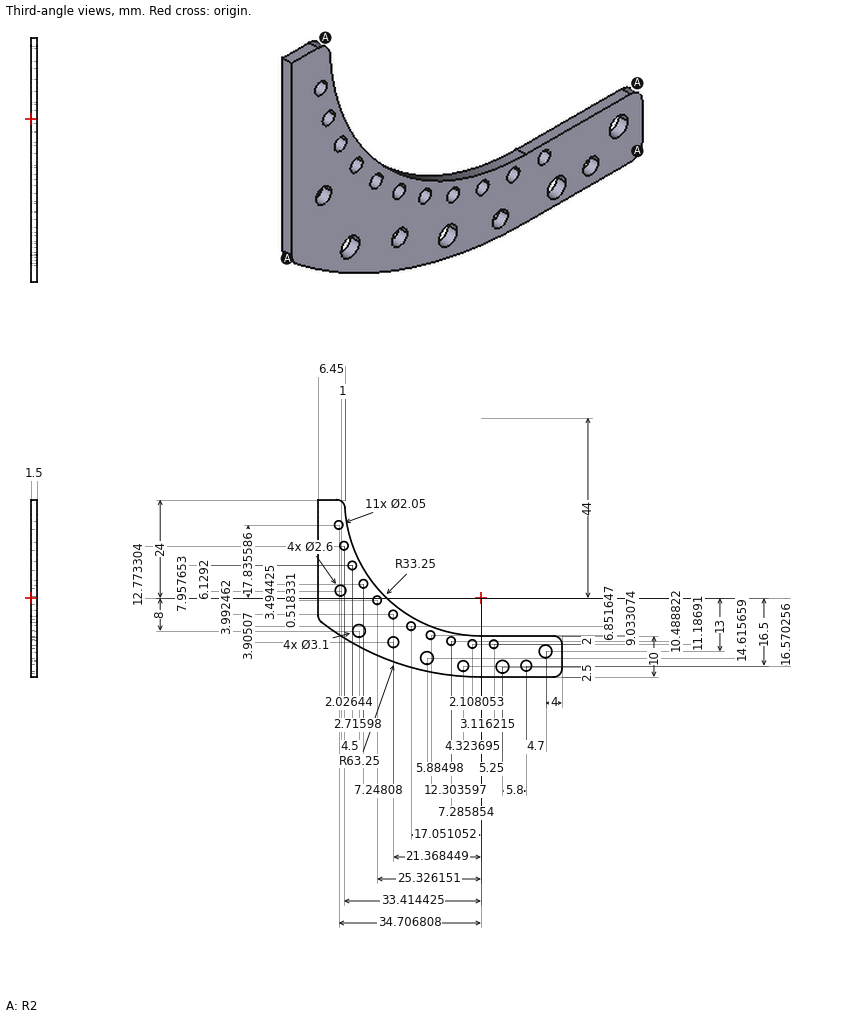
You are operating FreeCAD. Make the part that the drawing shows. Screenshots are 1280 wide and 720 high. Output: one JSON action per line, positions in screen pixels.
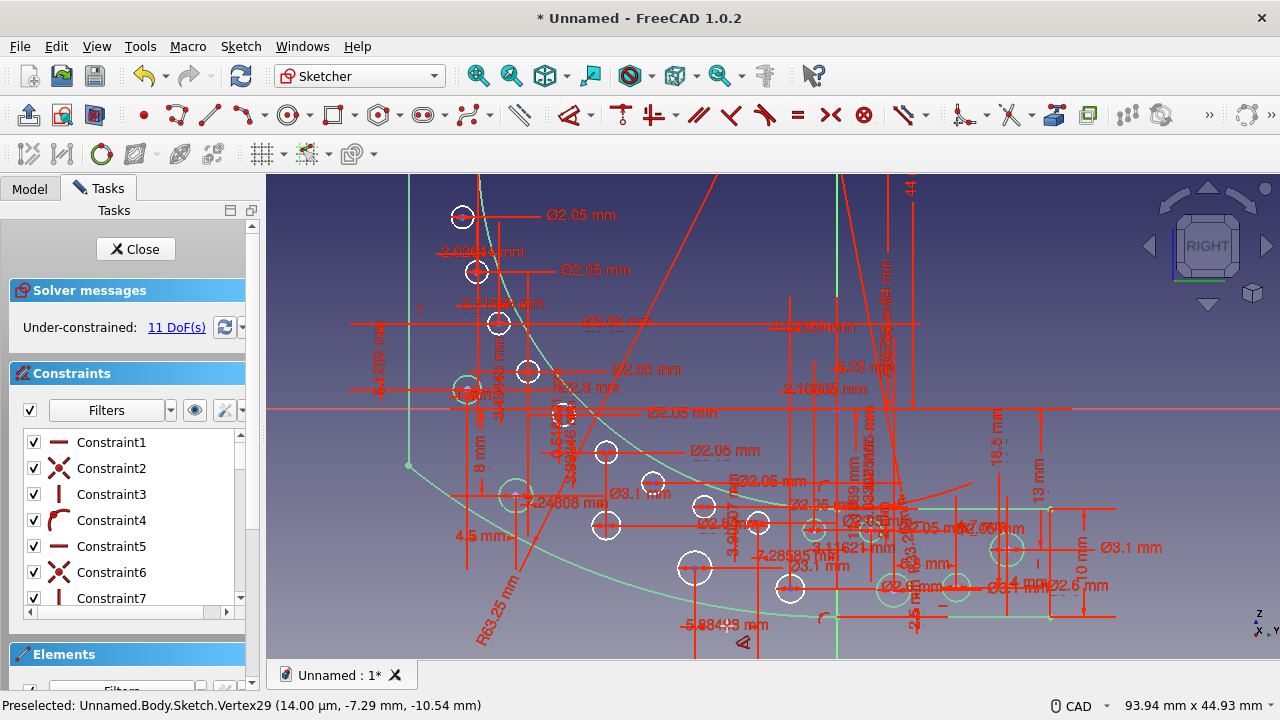
{"action": "left_click", "coordinate": [463, 217]}
{"action": "left_click", "coordinate": [736, 443]}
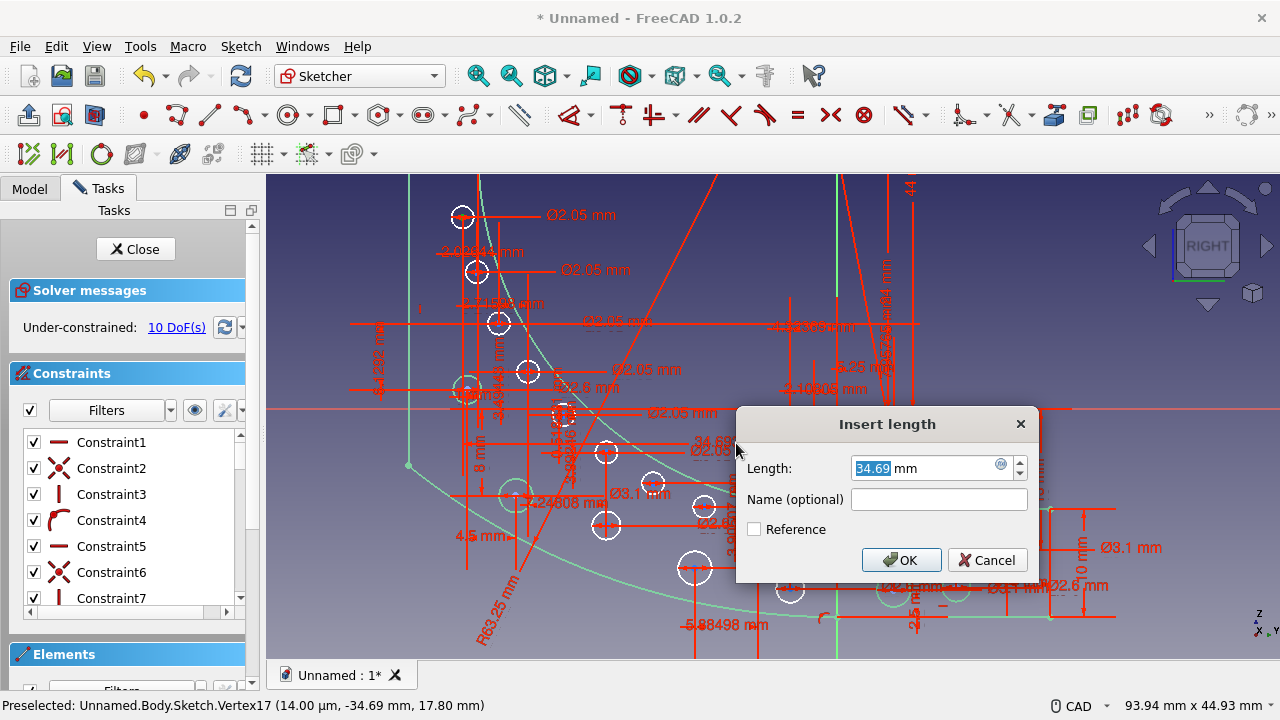
{"action": "type", "text": "34.706808"}
{"action": "key", "text": "Return"}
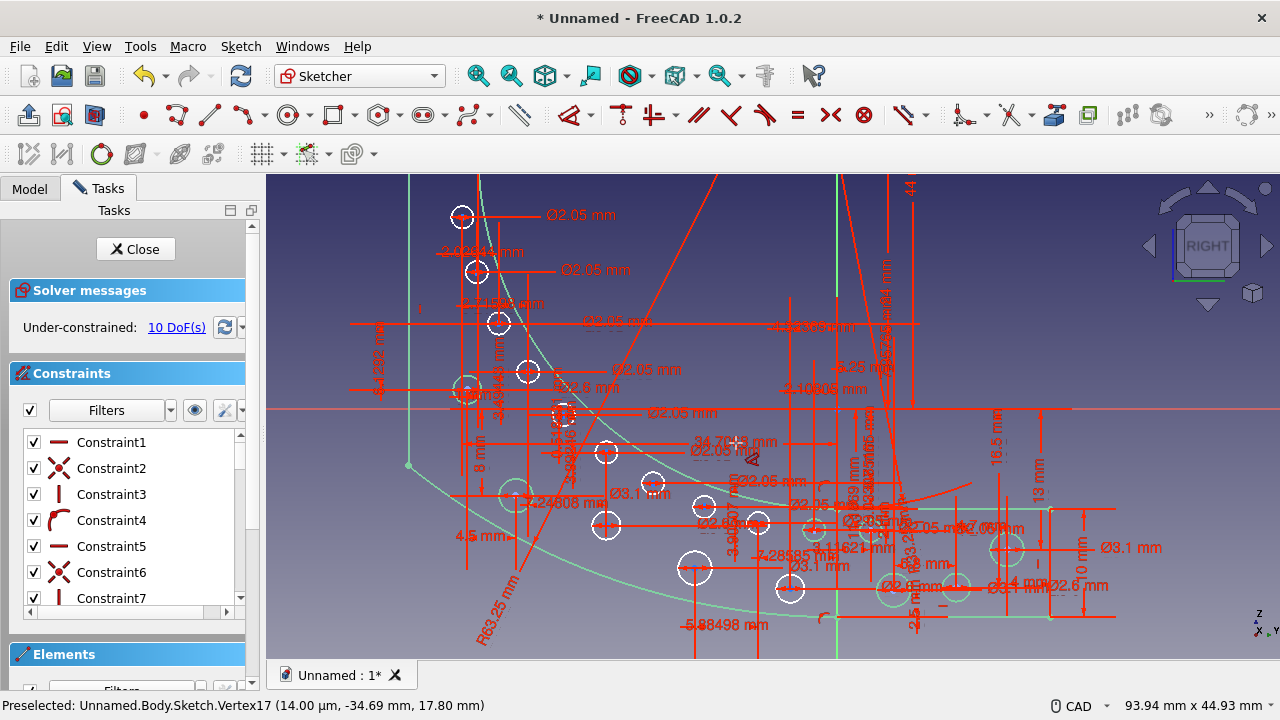
{"action": "left_click", "coordinate": [462, 217]}
{"action": "left_click", "coordinate": [428, 313]}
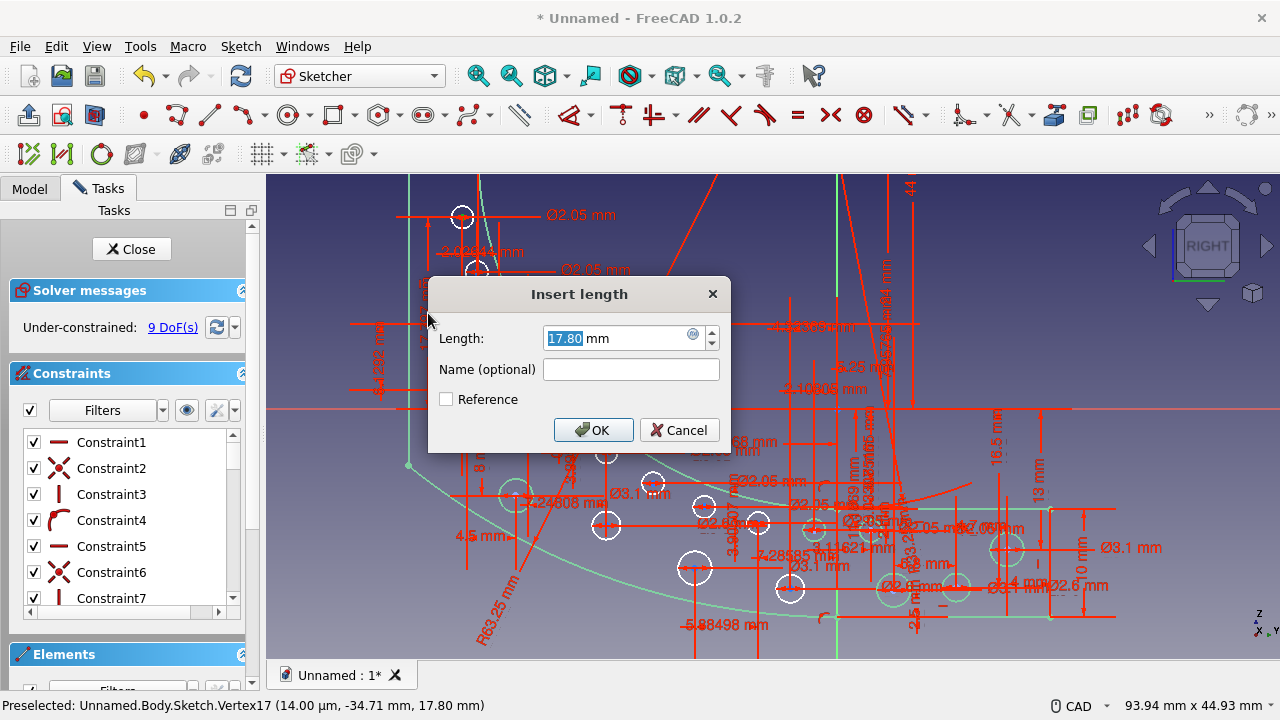
{"action": "type", "text": "17.835586"}
{"action": "key", "text": "Return"}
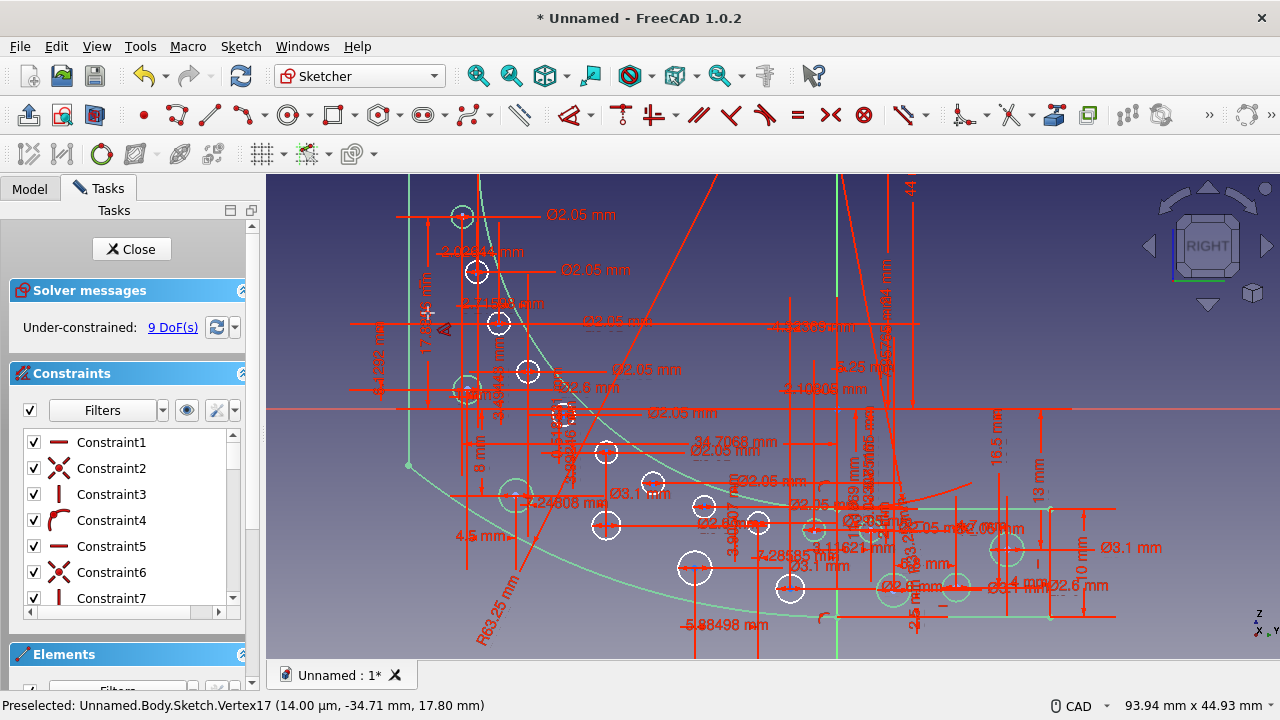
{"action": "left_click", "coordinate": [477, 272]}
{"action": "left_click", "coordinate": [657, 238]}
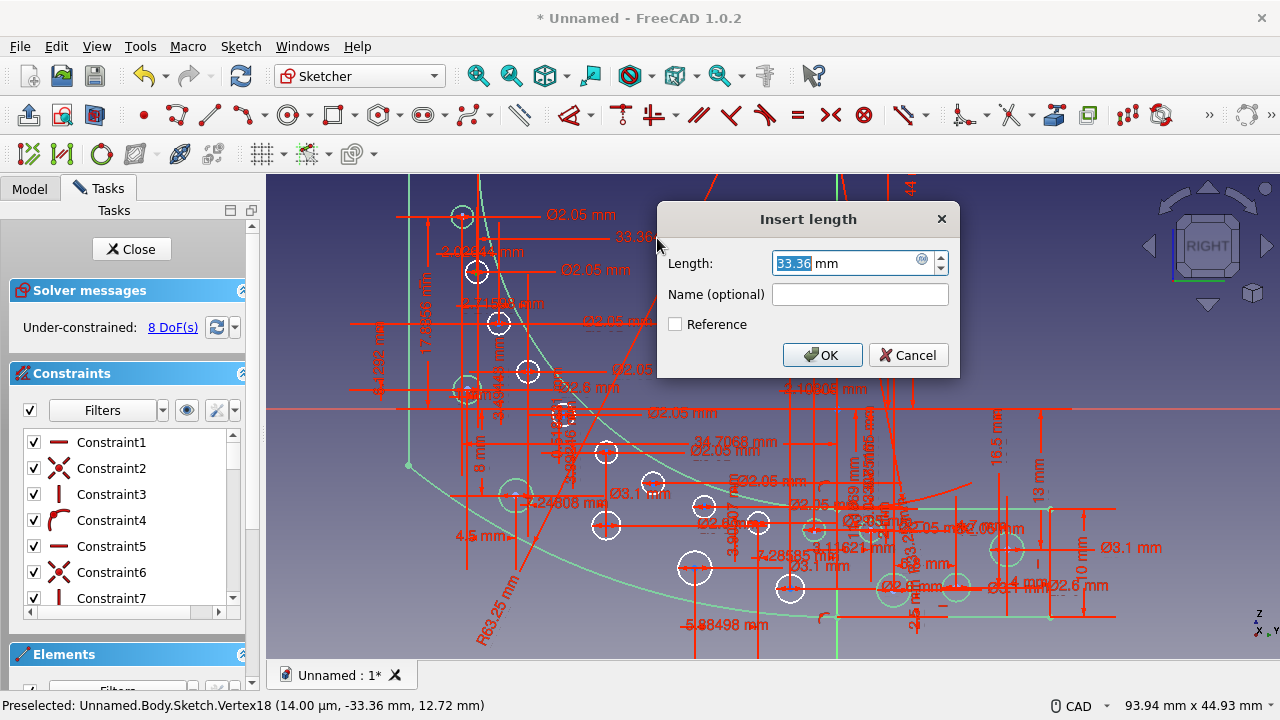
{"action": "type", "text": "33.414425"}
{"action": "key", "text": "Return"}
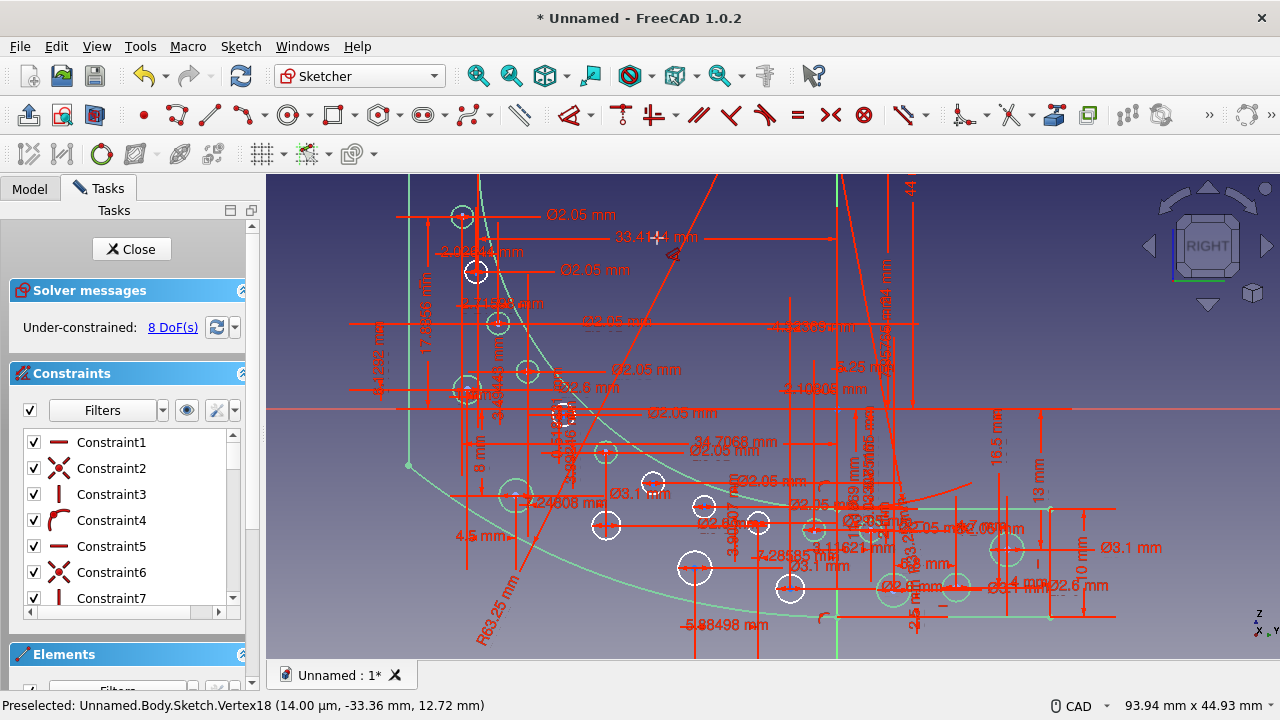
{"action": "left_click", "coordinate": [476, 272]}
{"action": "left_click", "coordinate": [895, 309]}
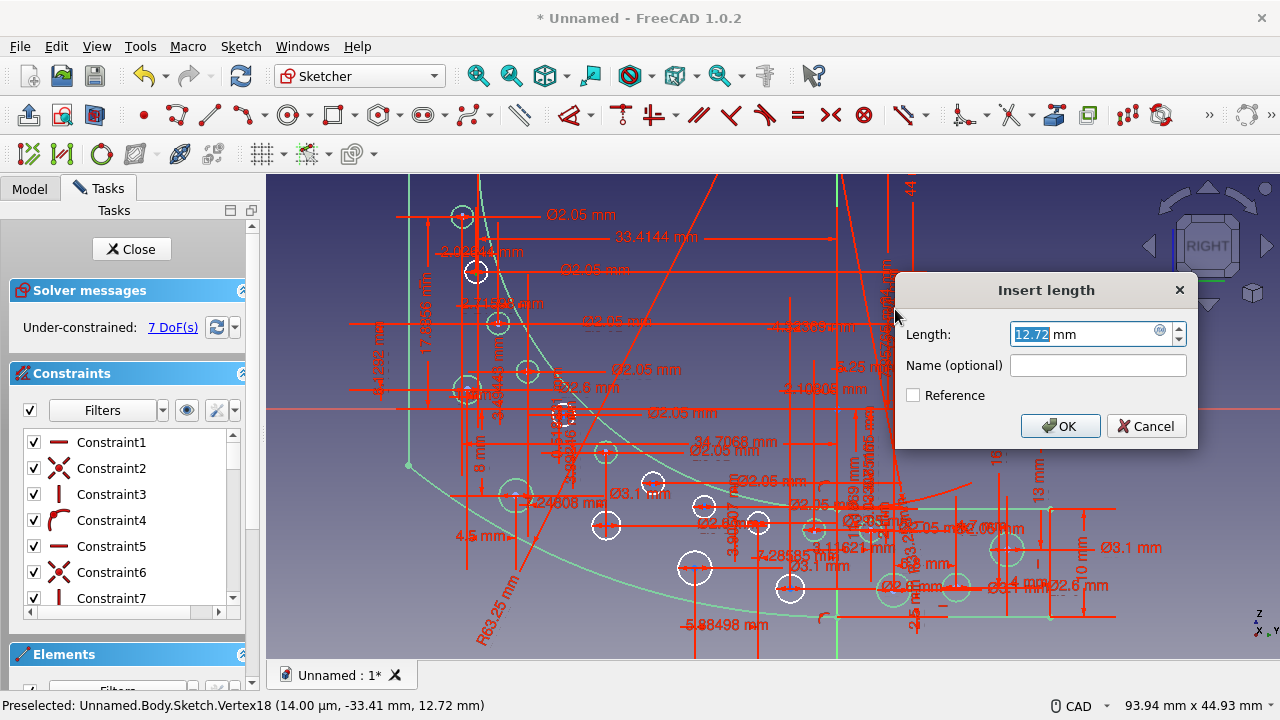
{"action": "type", "text": "12.773304"}
{"action": "key", "text": "Return"}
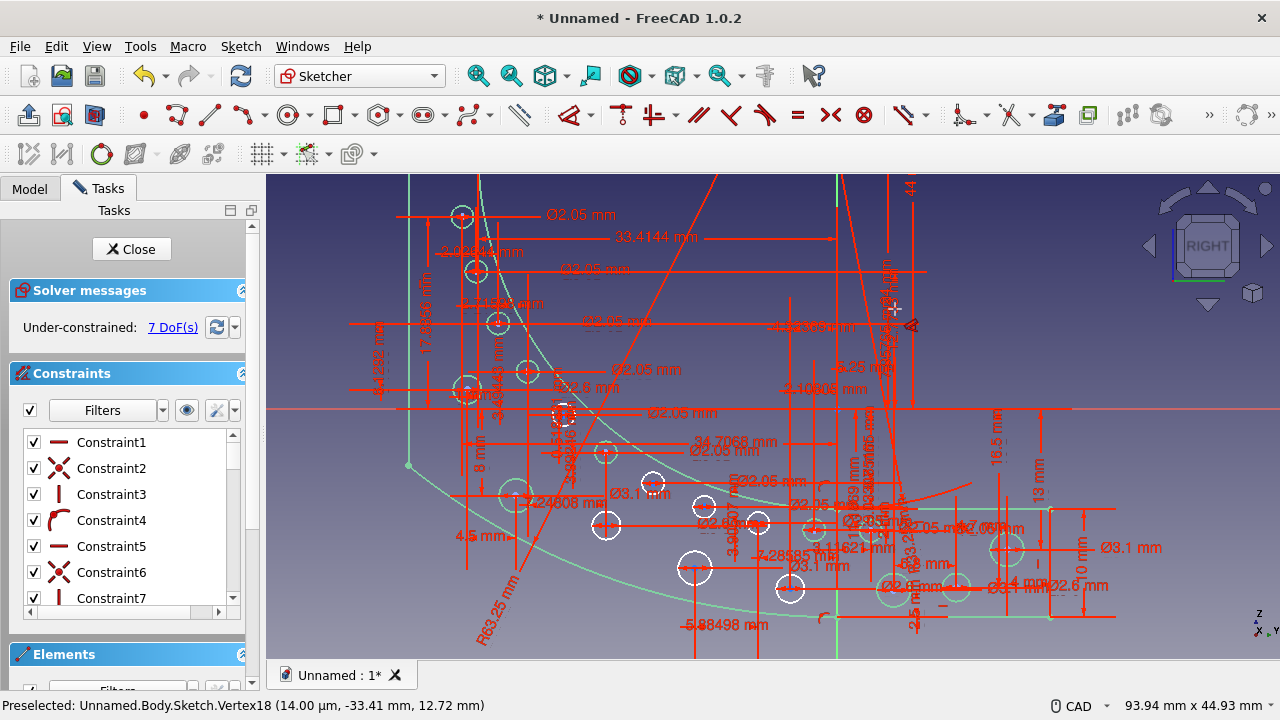
{"action": "left_click", "coordinate": [564, 415]}
{"action": "left_click", "coordinate": [700, 375]}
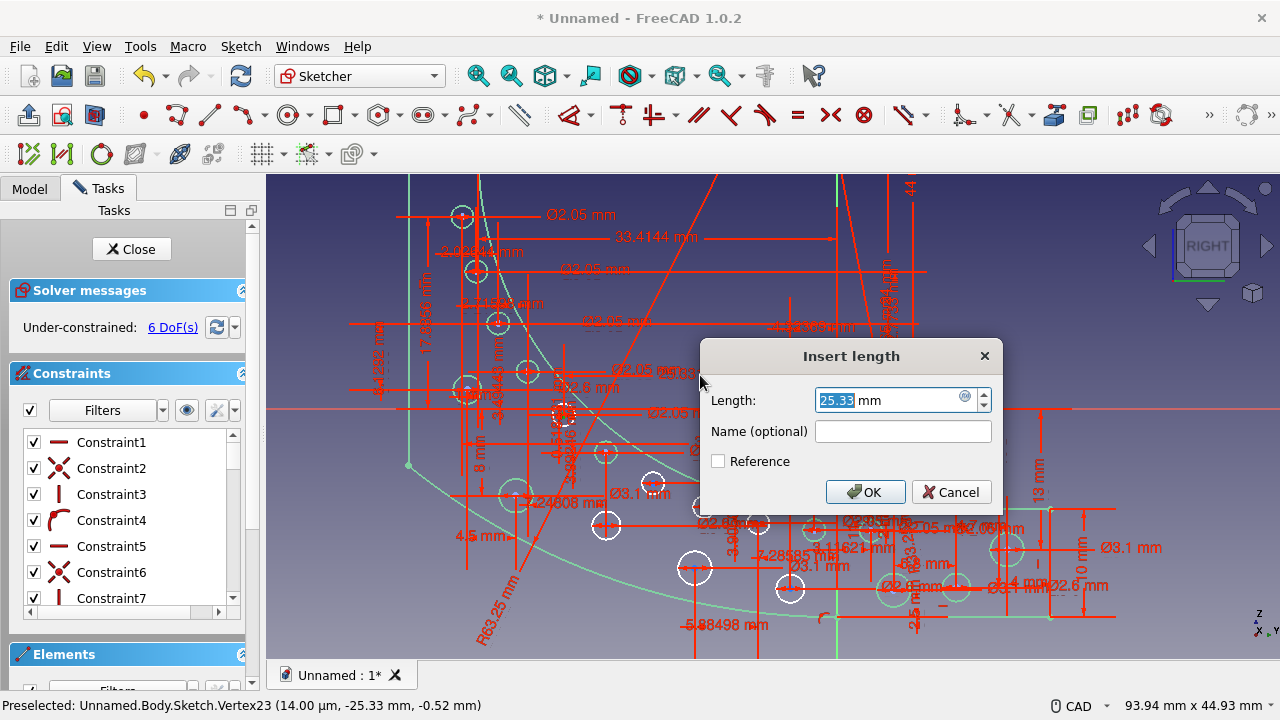
{"action": "type", "text": "25.326151"}
{"action": "key", "text": "Return"}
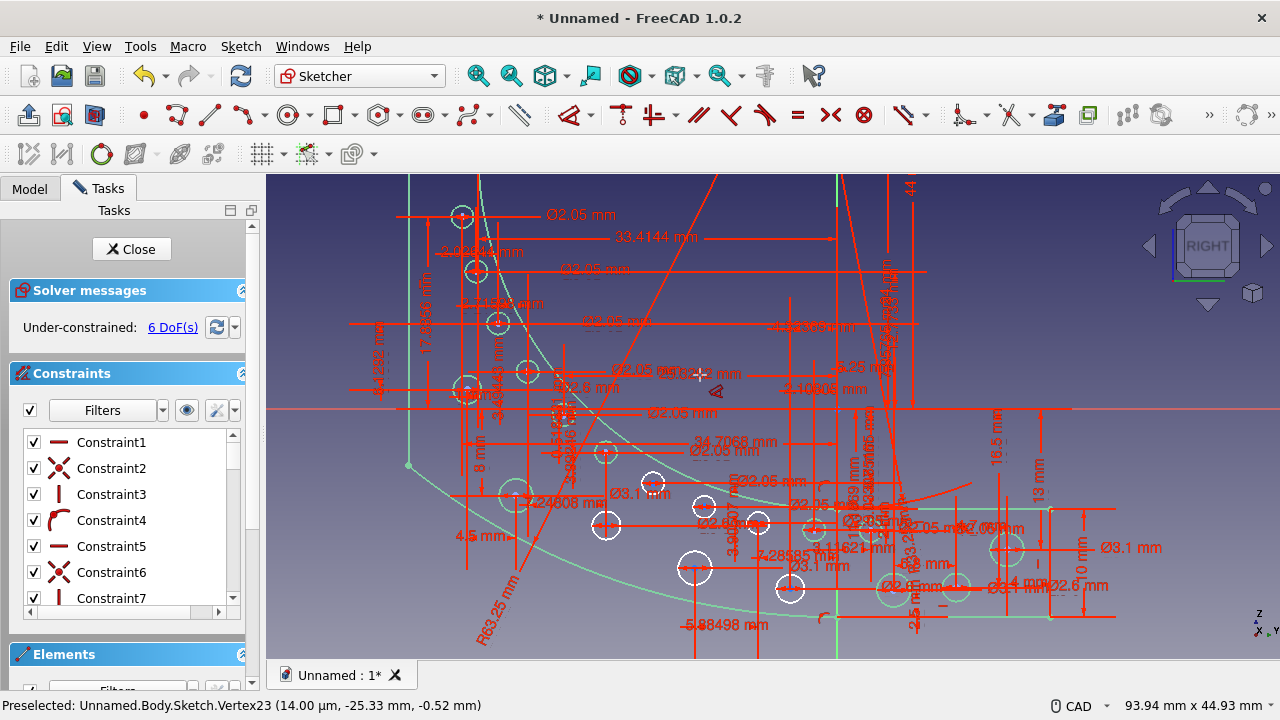
{"action": "left_click", "coordinate": [653, 483]}
{"action": "left_click", "coordinate": [681, 541]}